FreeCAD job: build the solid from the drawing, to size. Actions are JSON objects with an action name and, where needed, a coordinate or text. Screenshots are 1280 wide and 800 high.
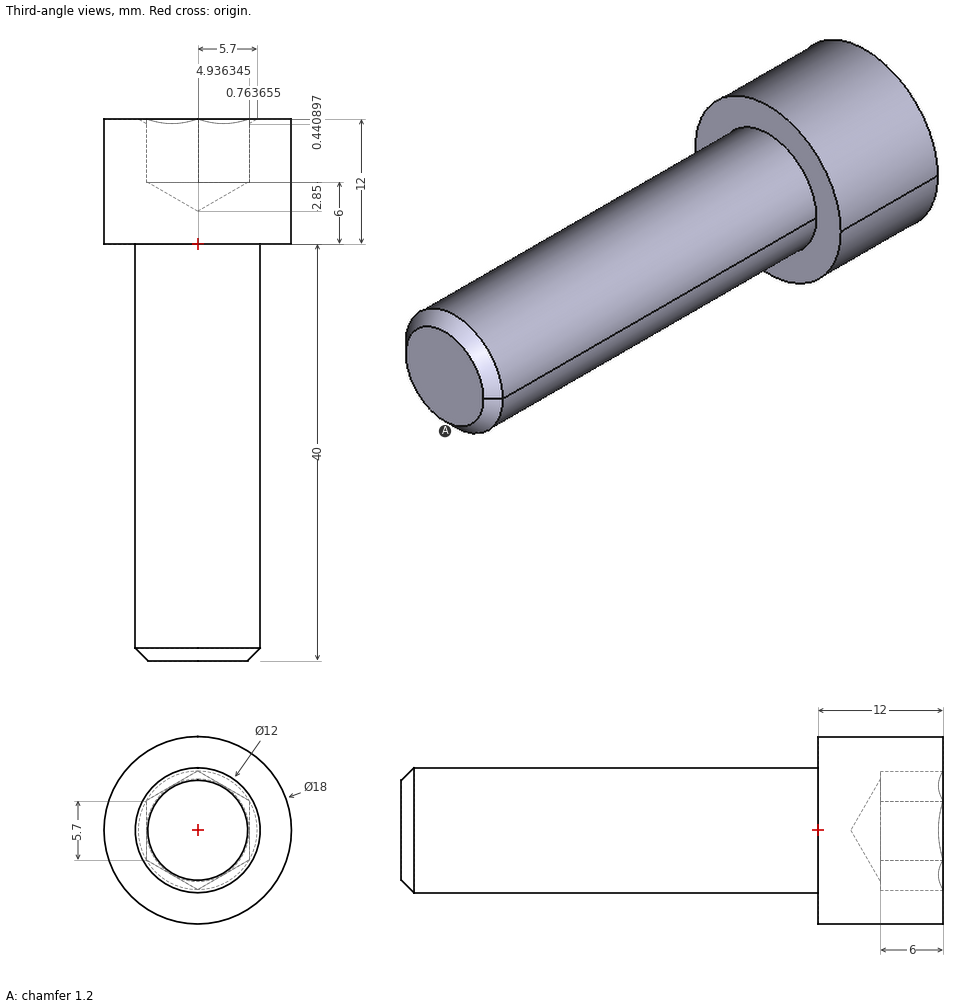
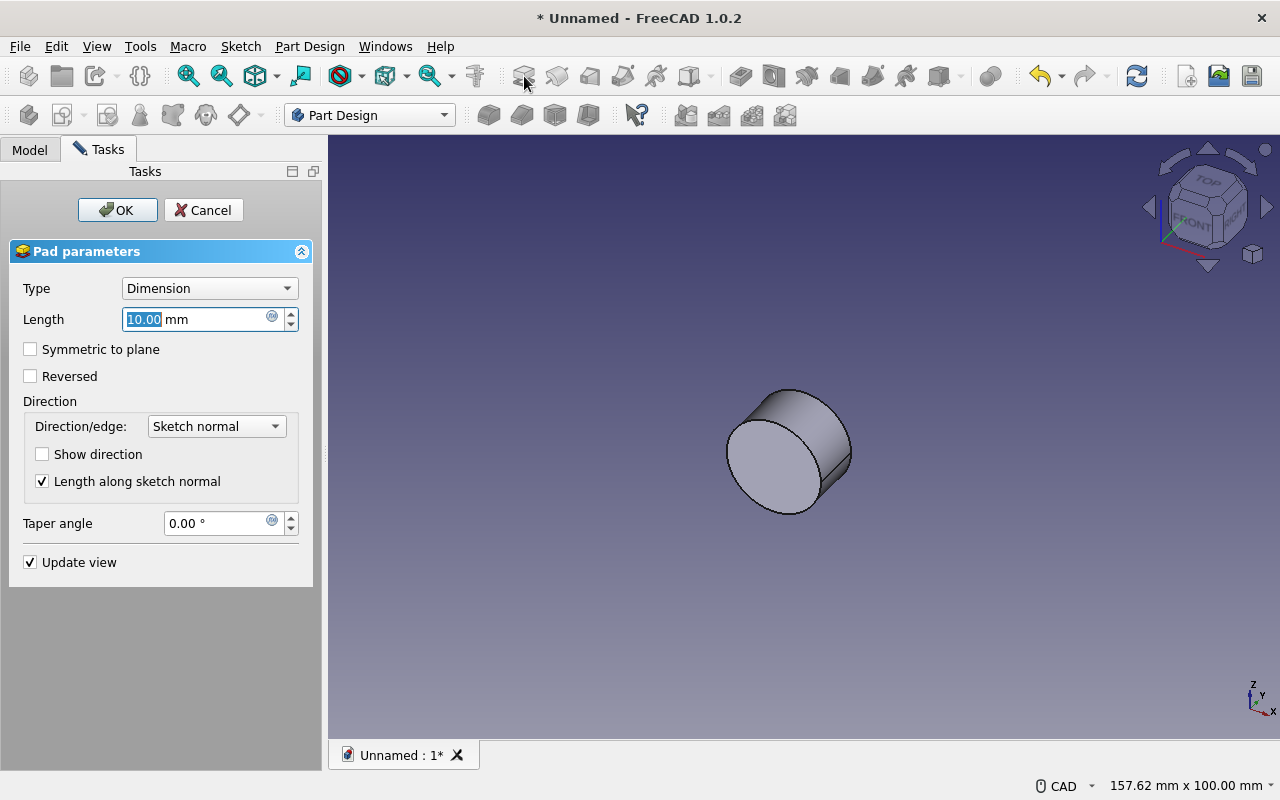
{"action": "type", "text": "12"}
{"action": "key", "text": "Tab"}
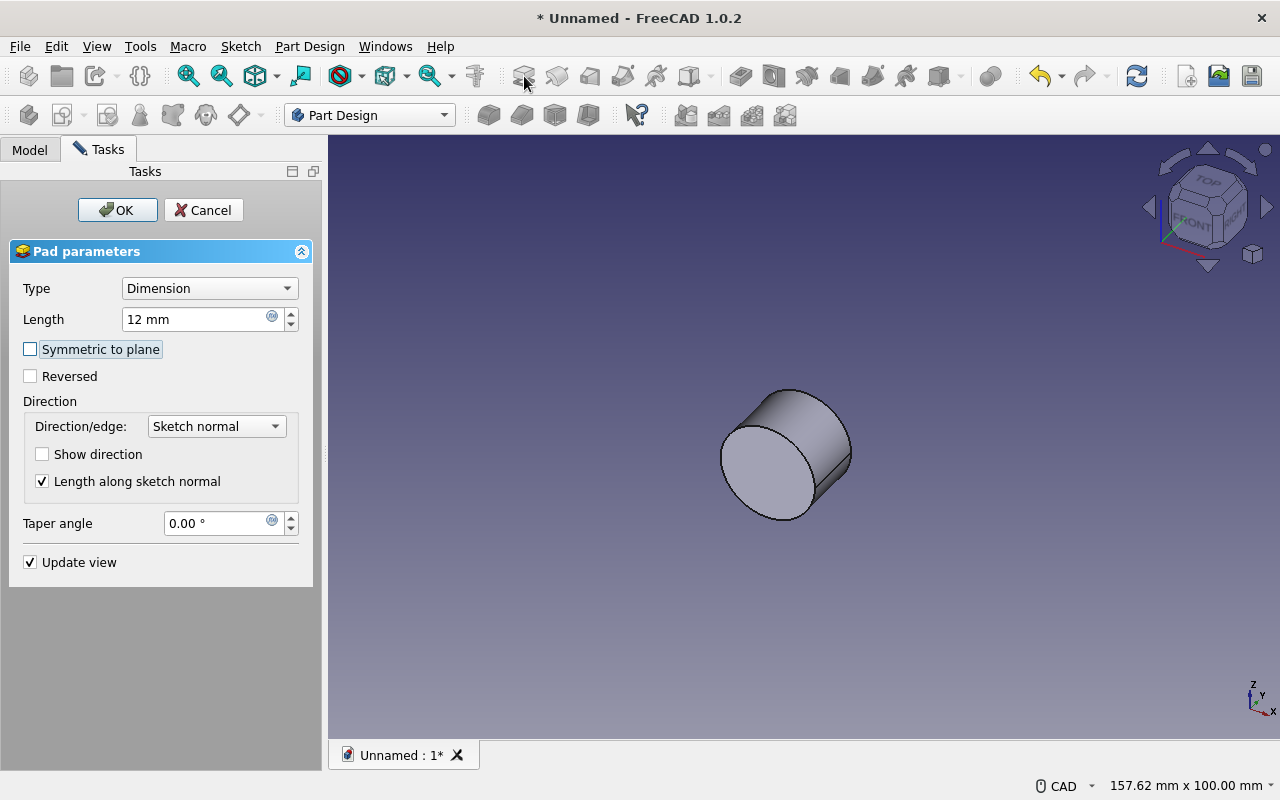
{"action": "left_click", "coordinate": [31, 376]}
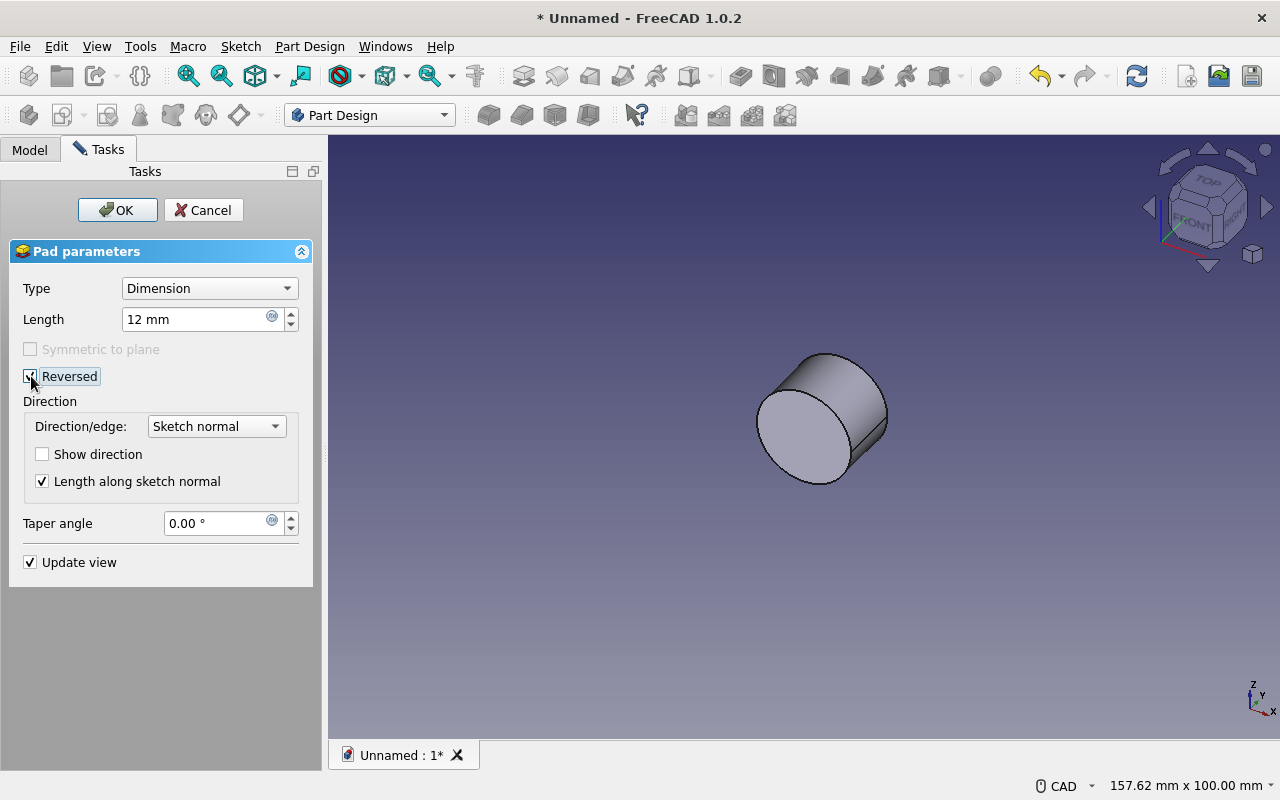
{"action": "left_click", "coordinate": [118, 210]}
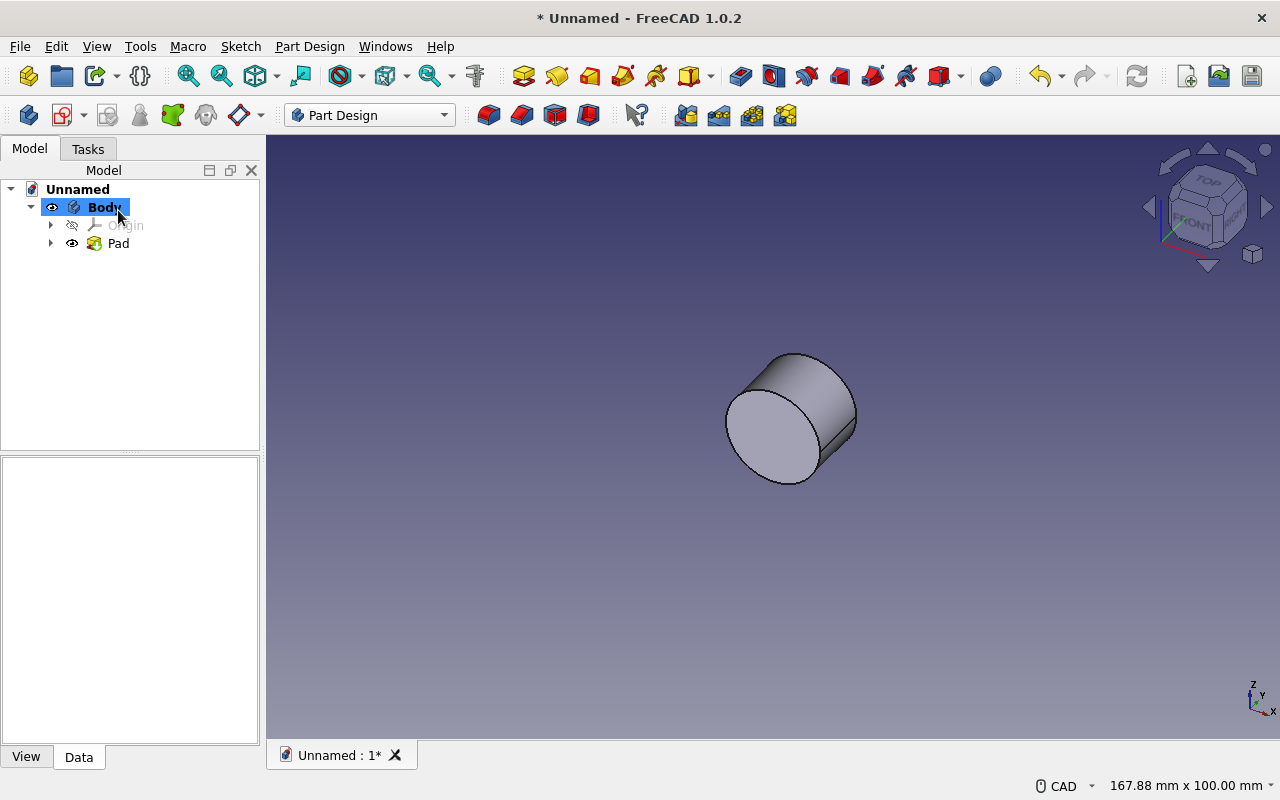
{"action": "left_click", "coordinate": [189, 76]}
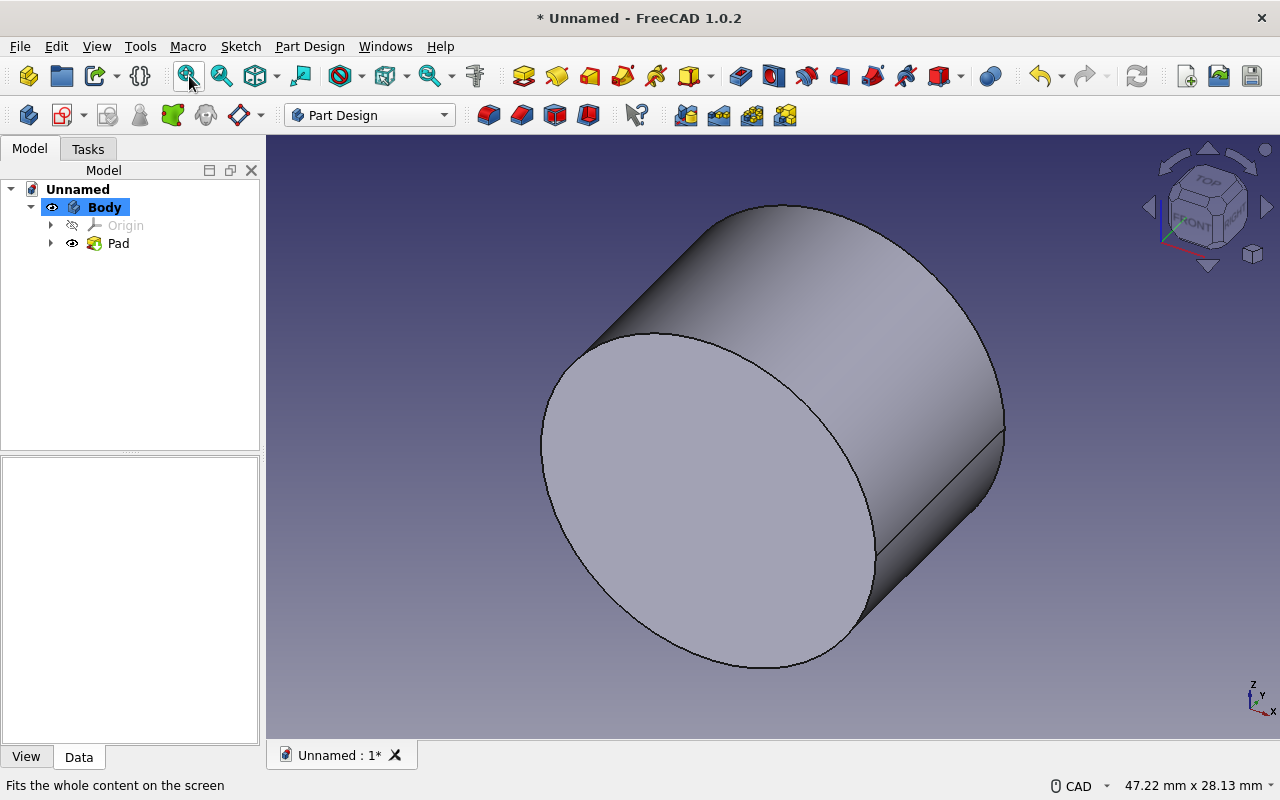
{"action": "left_click", "coordinate": [62, 116]}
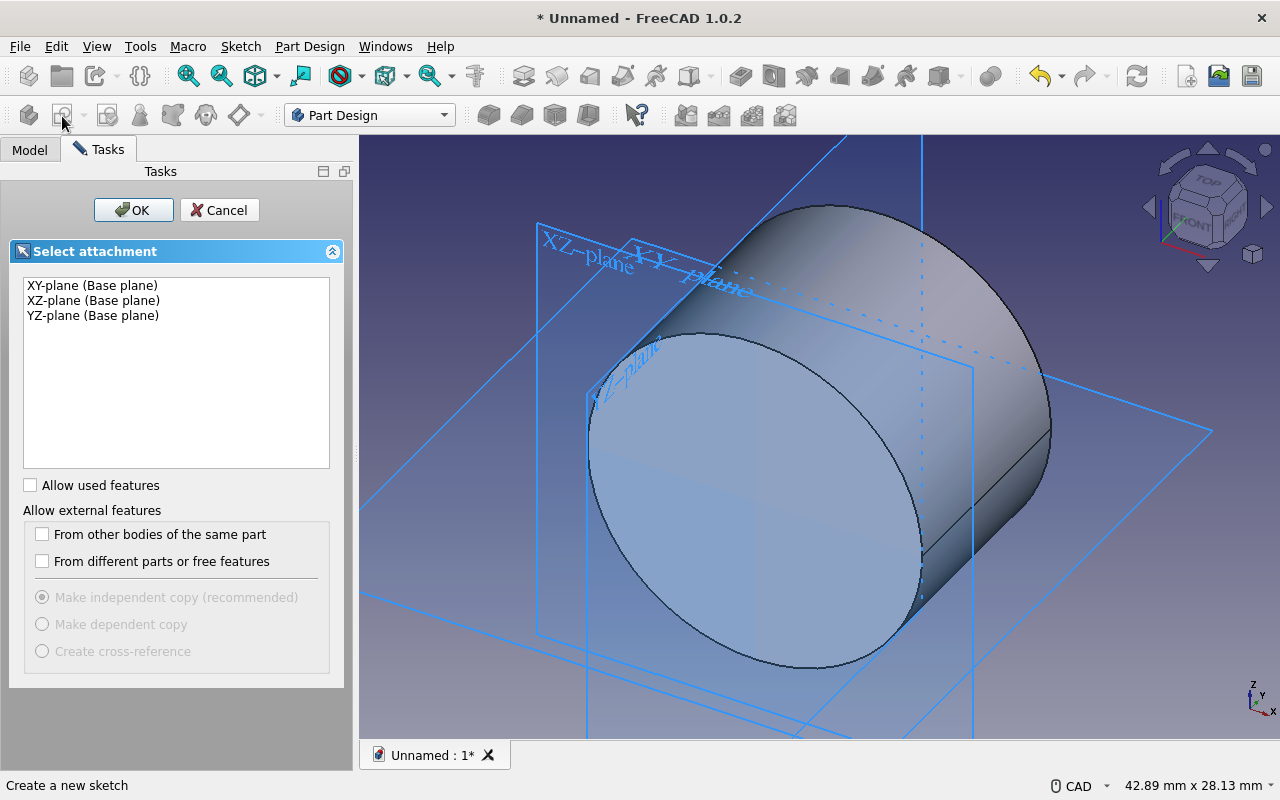
{"action": "left_click", "coordinate": [84, 300]}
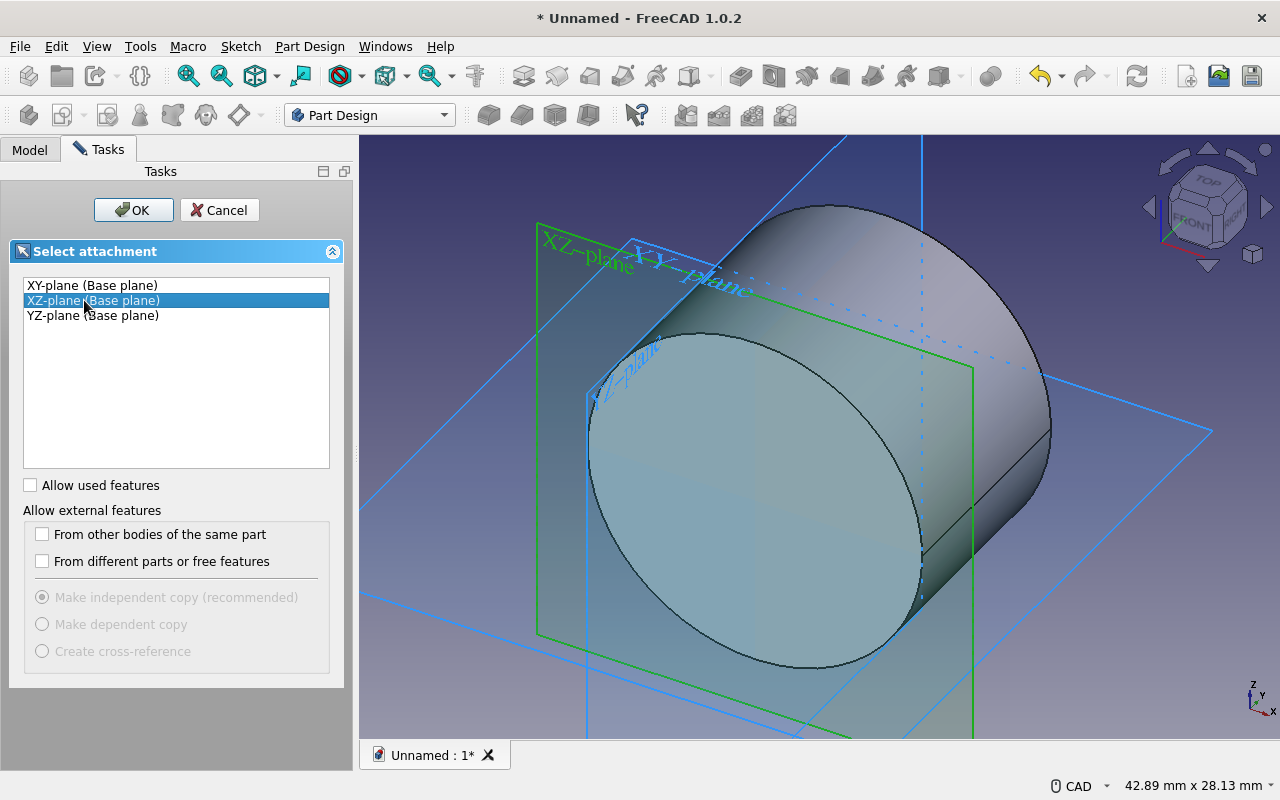
{"action": "left_click", "coordinate": [134, 210]}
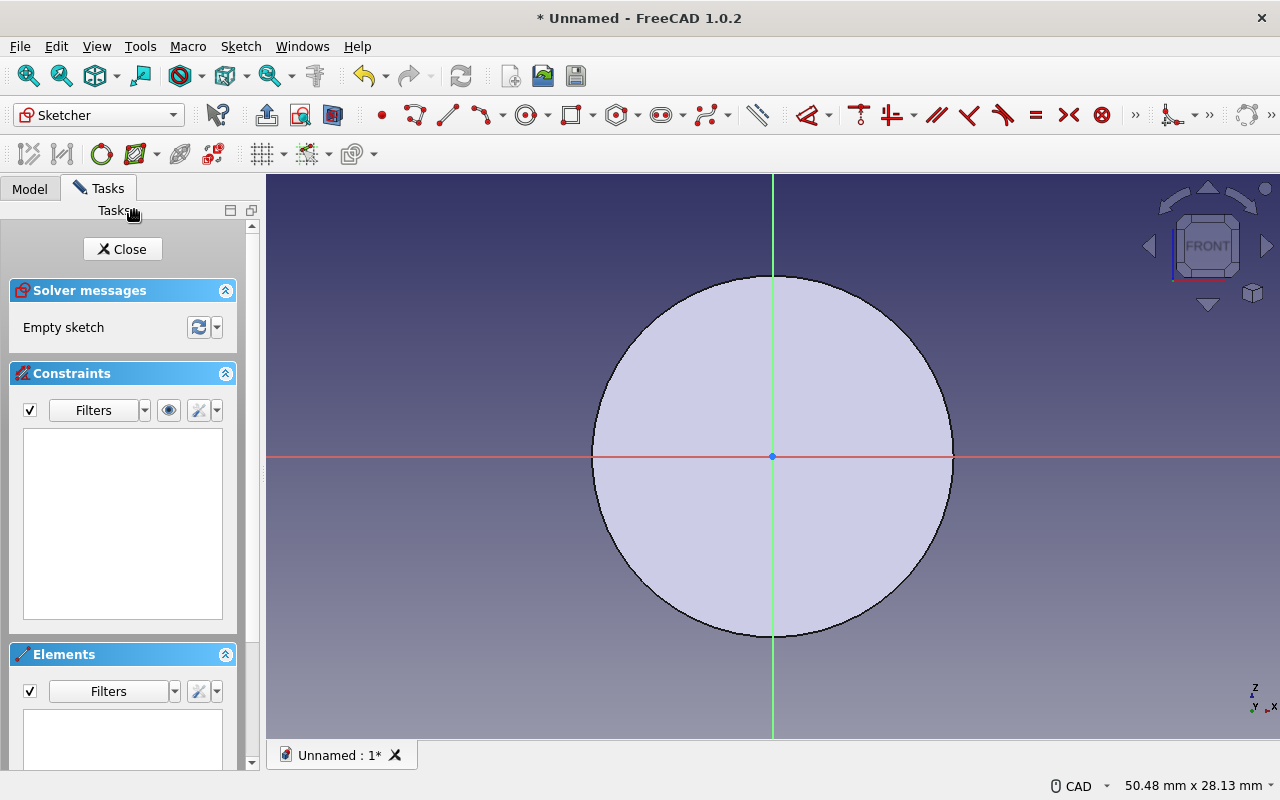
{"action": "scroll", "coordinate": [912, 457], "scroll_direction": "up", "scroll_amount": 2}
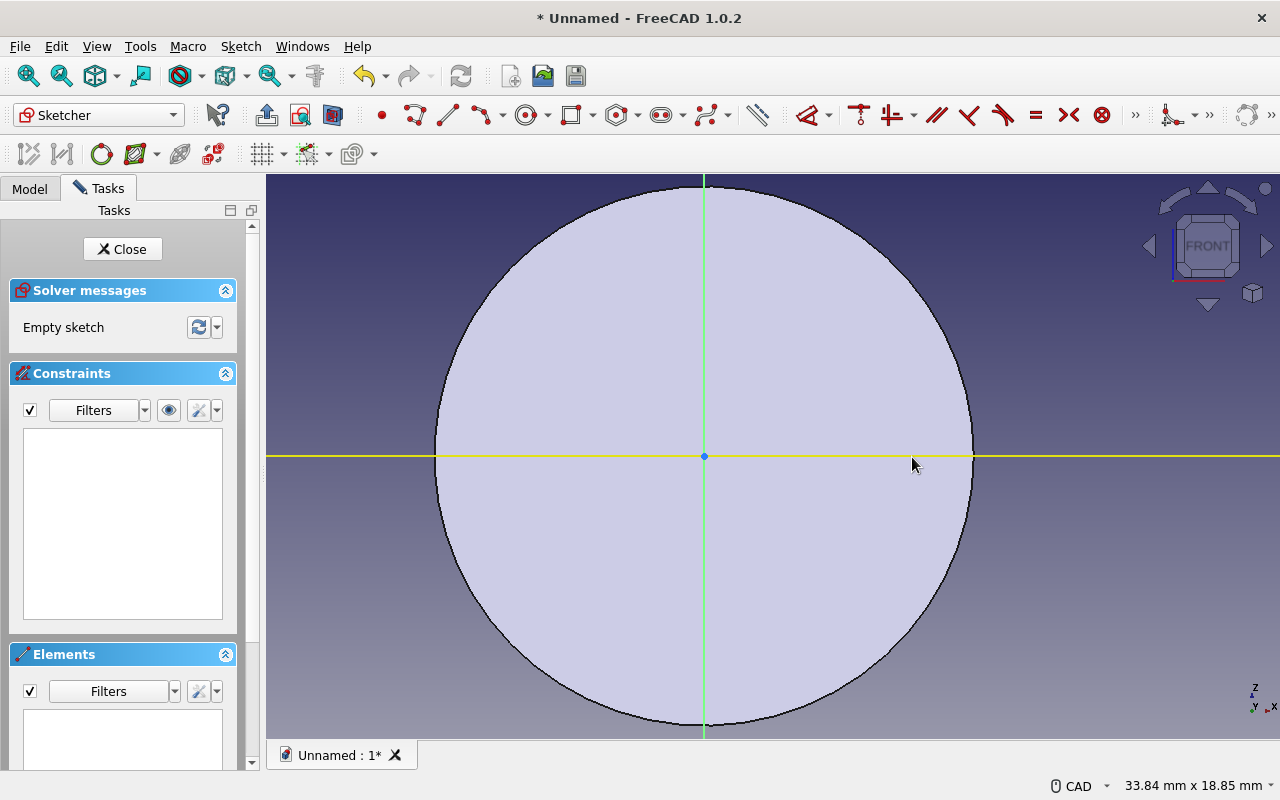
{"action": "left_click", "coordinate": [526, 116]}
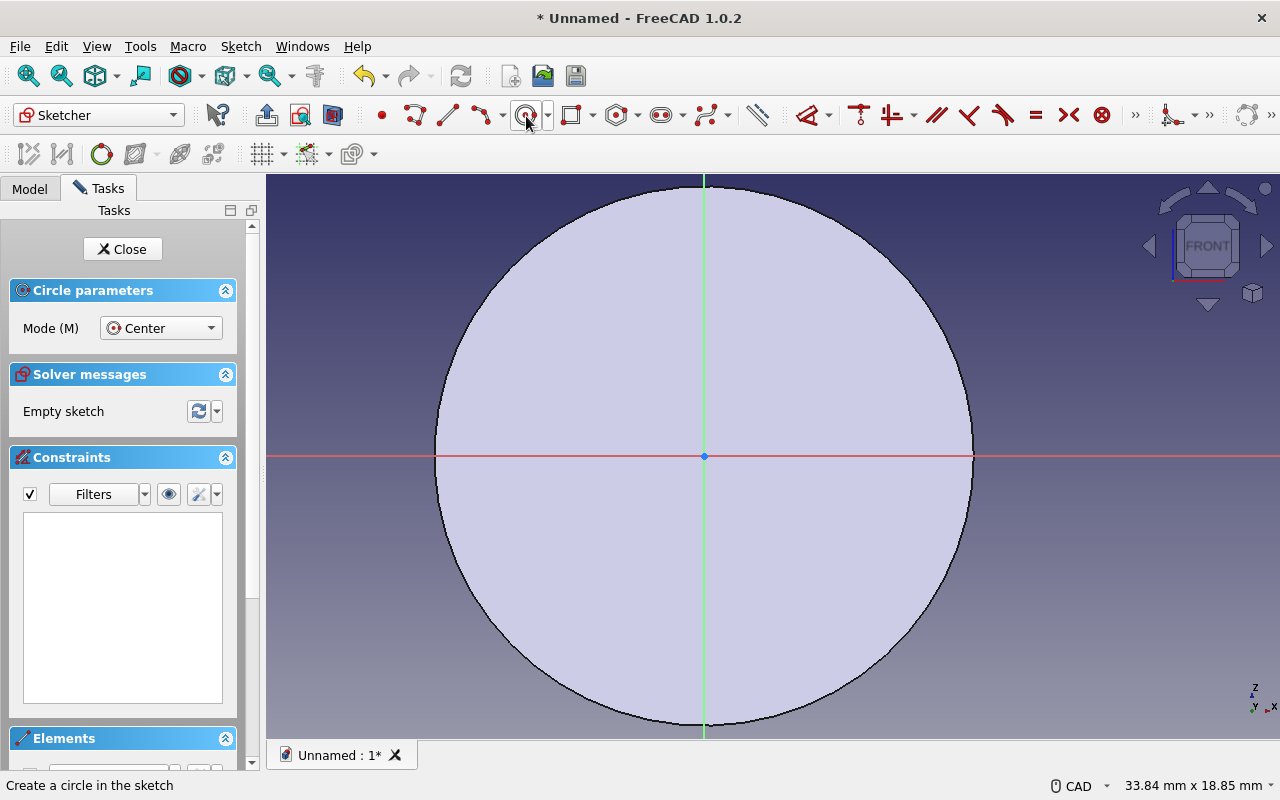
{"action": "left_click", "coordinate": [704, 456]}
{"action": "mouse_move", "coordinate": [831, 329]}